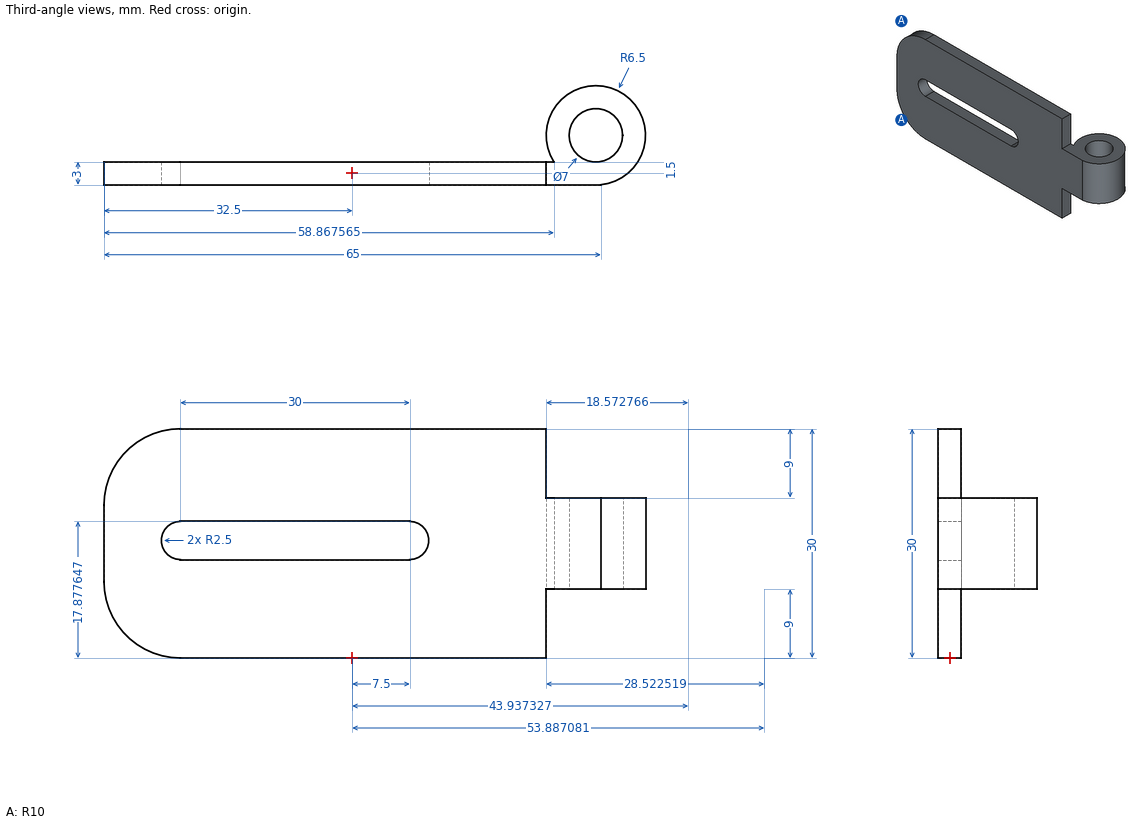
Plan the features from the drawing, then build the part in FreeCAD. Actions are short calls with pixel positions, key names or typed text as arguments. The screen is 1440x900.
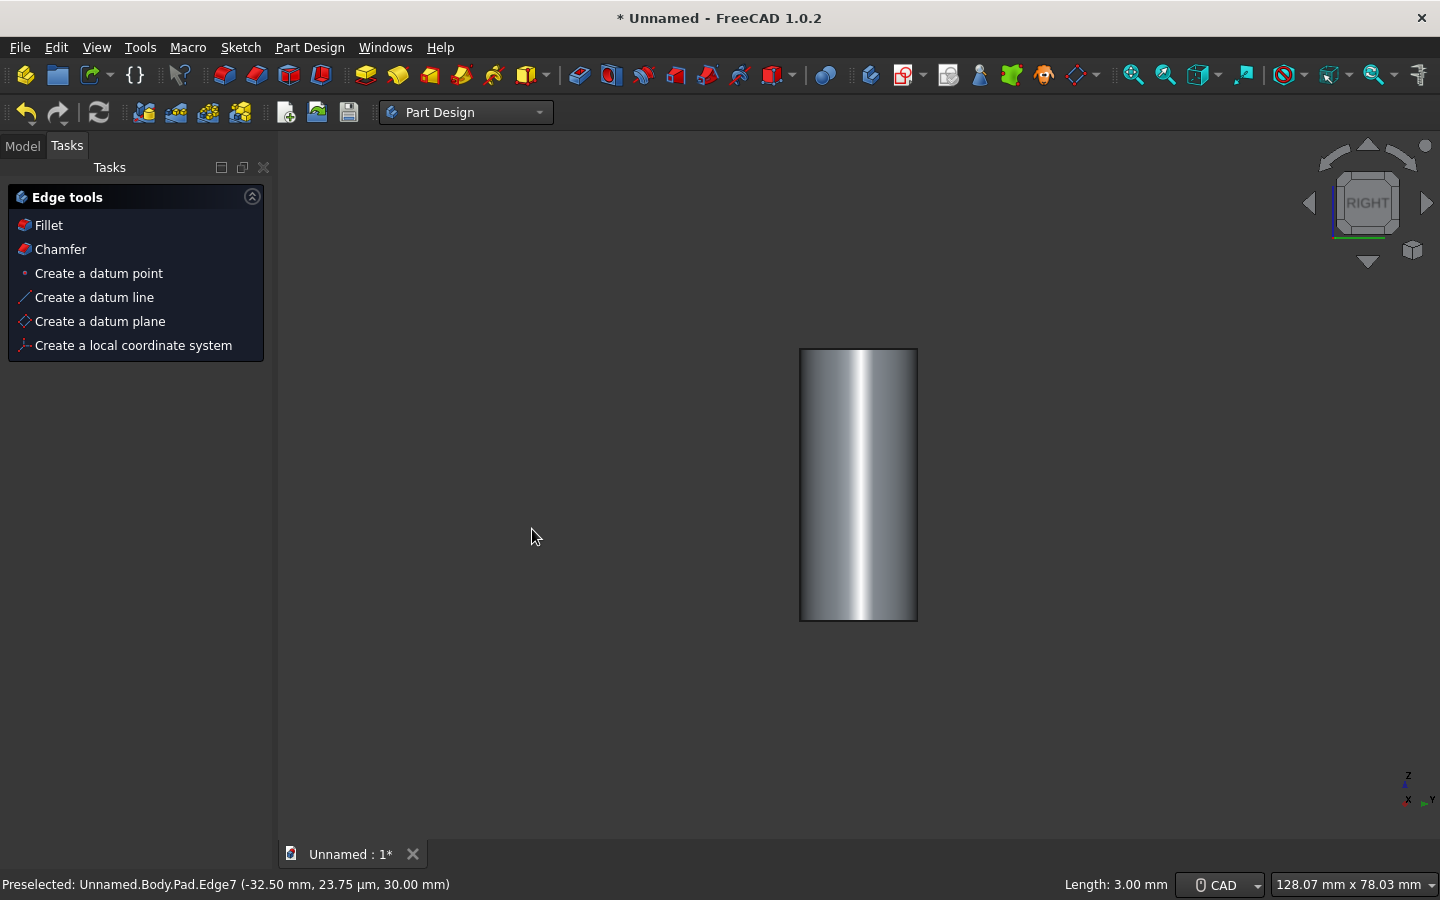
click(1134, 76)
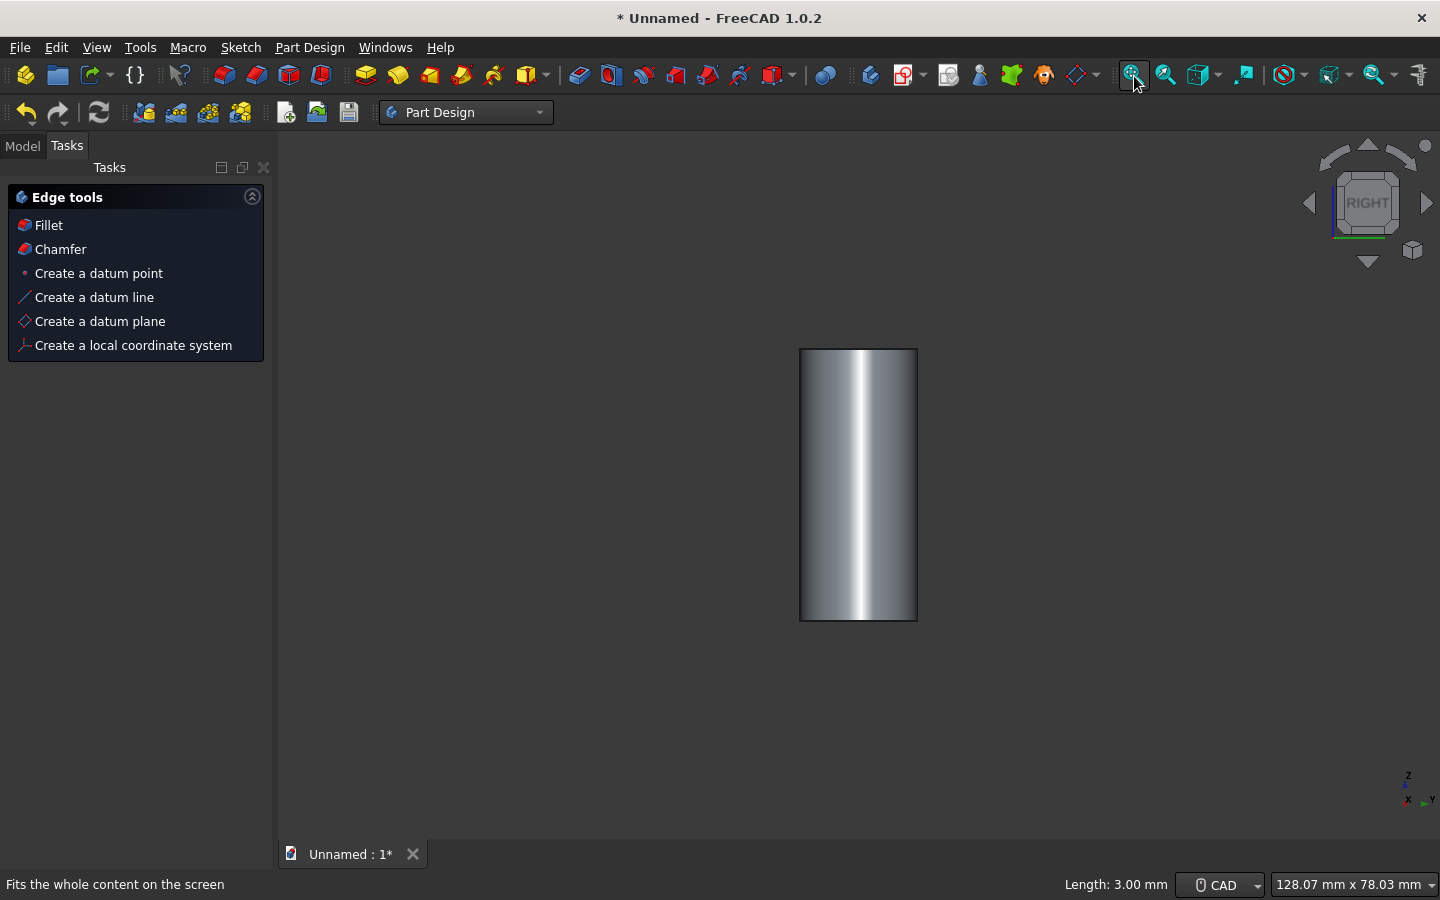
key(5)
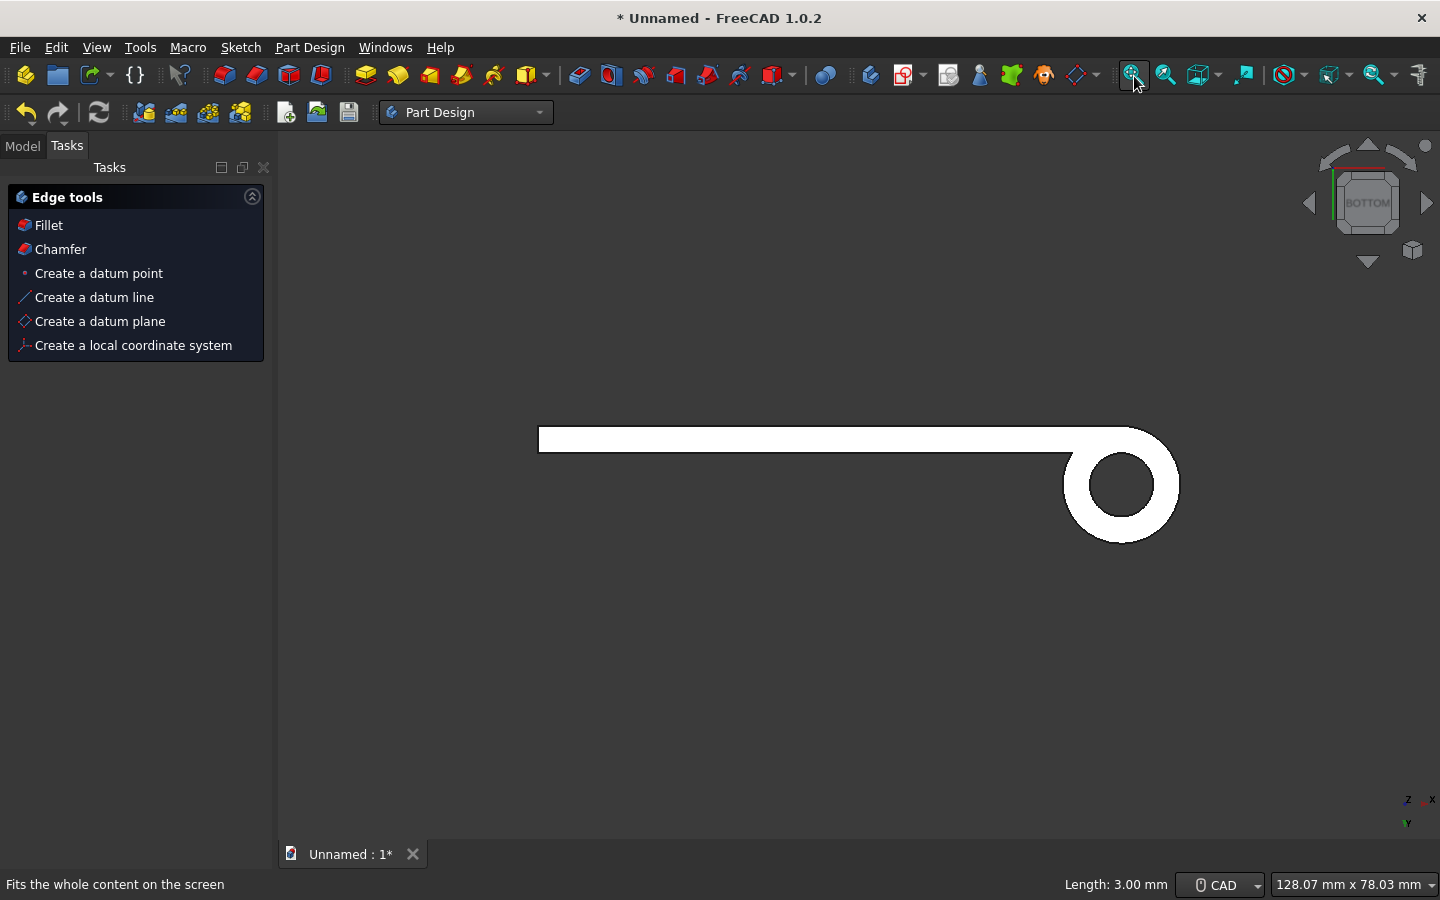
click(538, 439, ctrl)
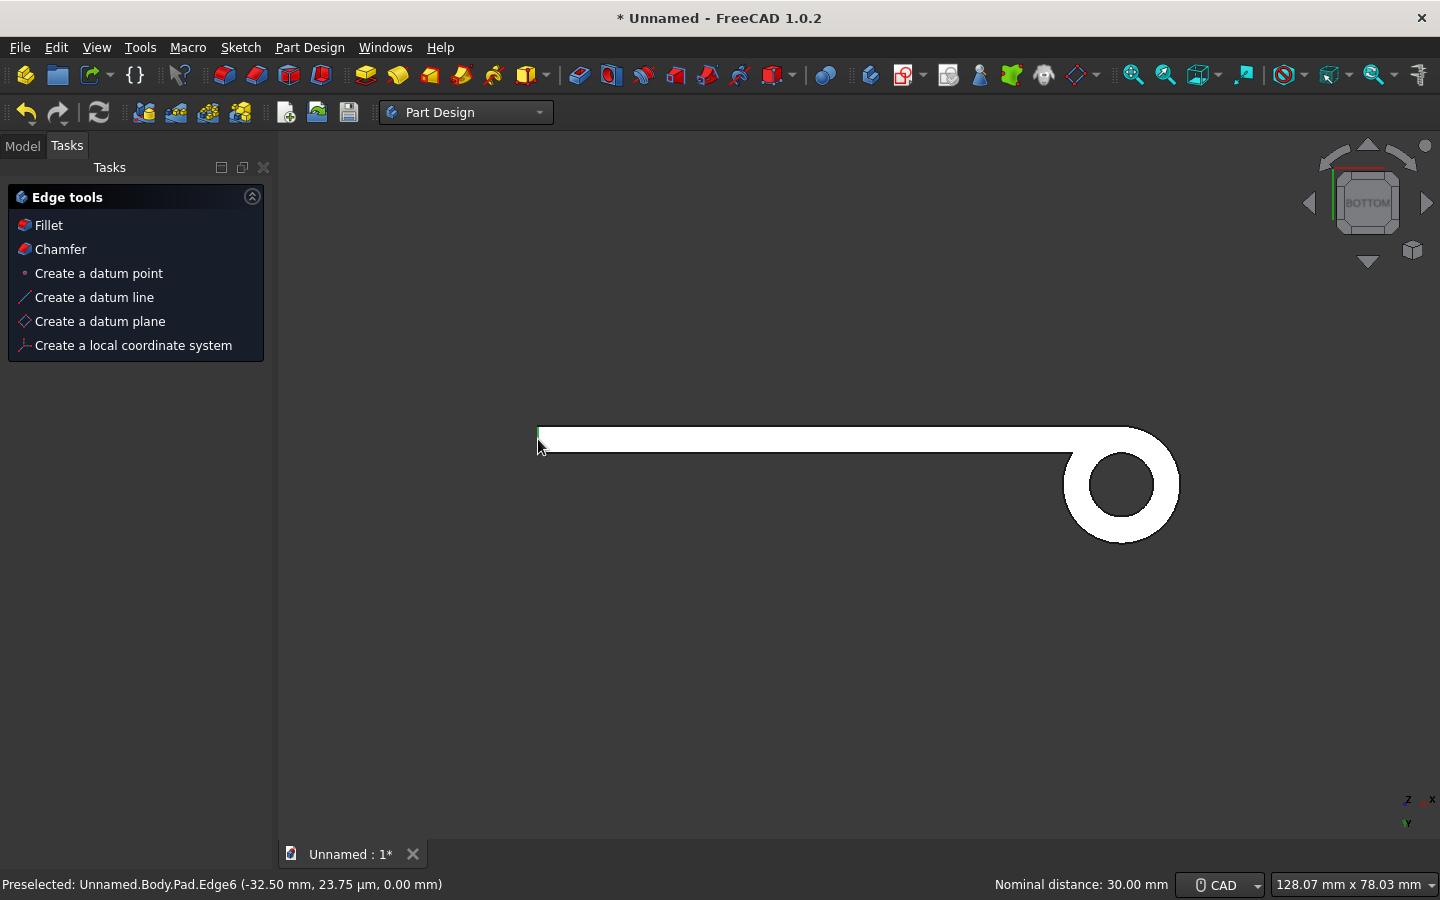
click(226, 76)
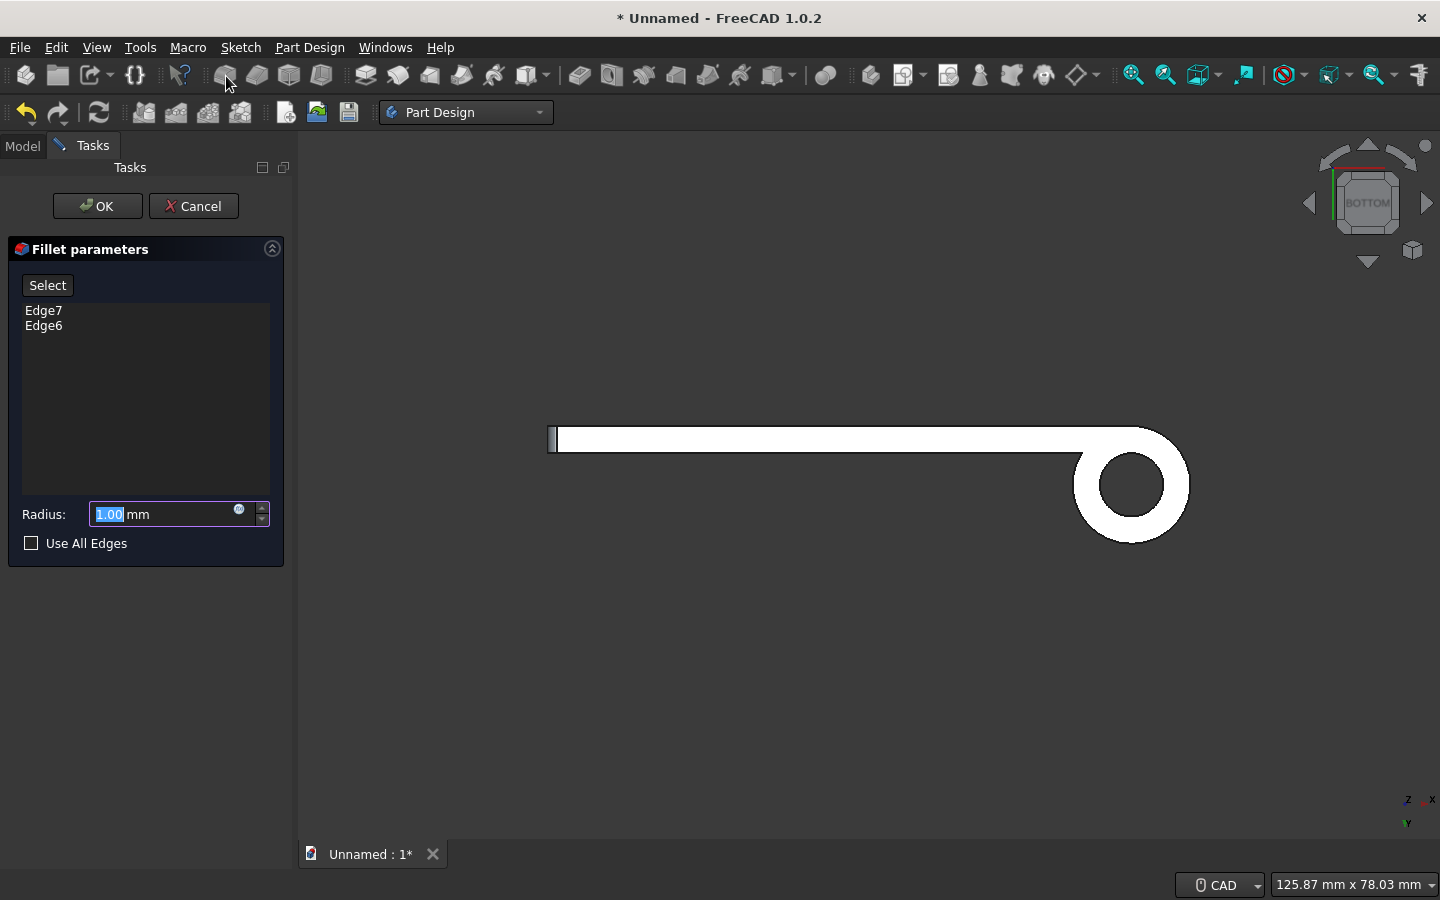
text(10)
key(Tab)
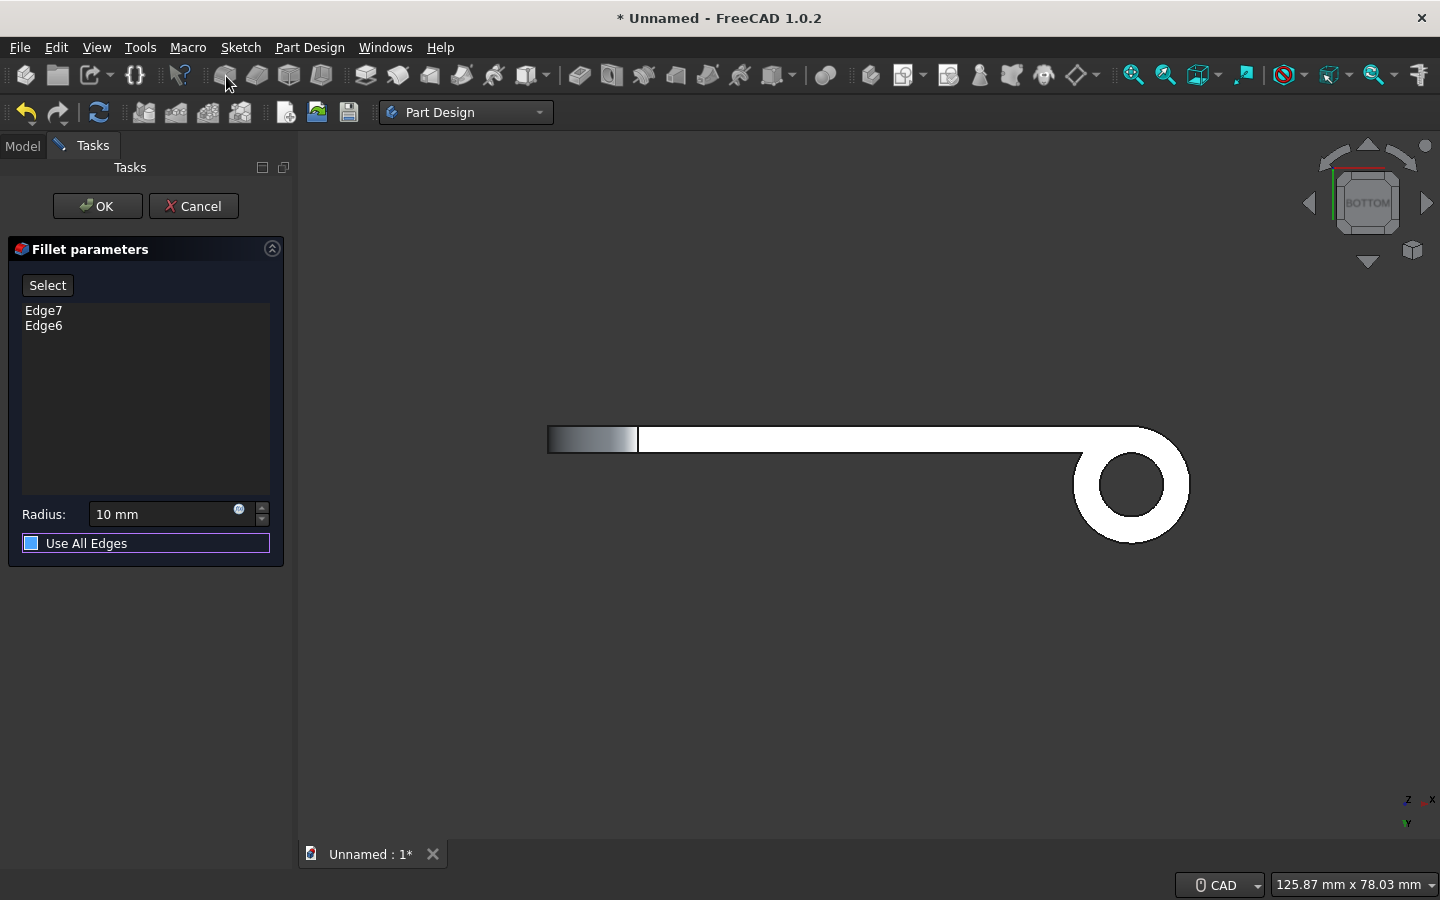
click(98, 206)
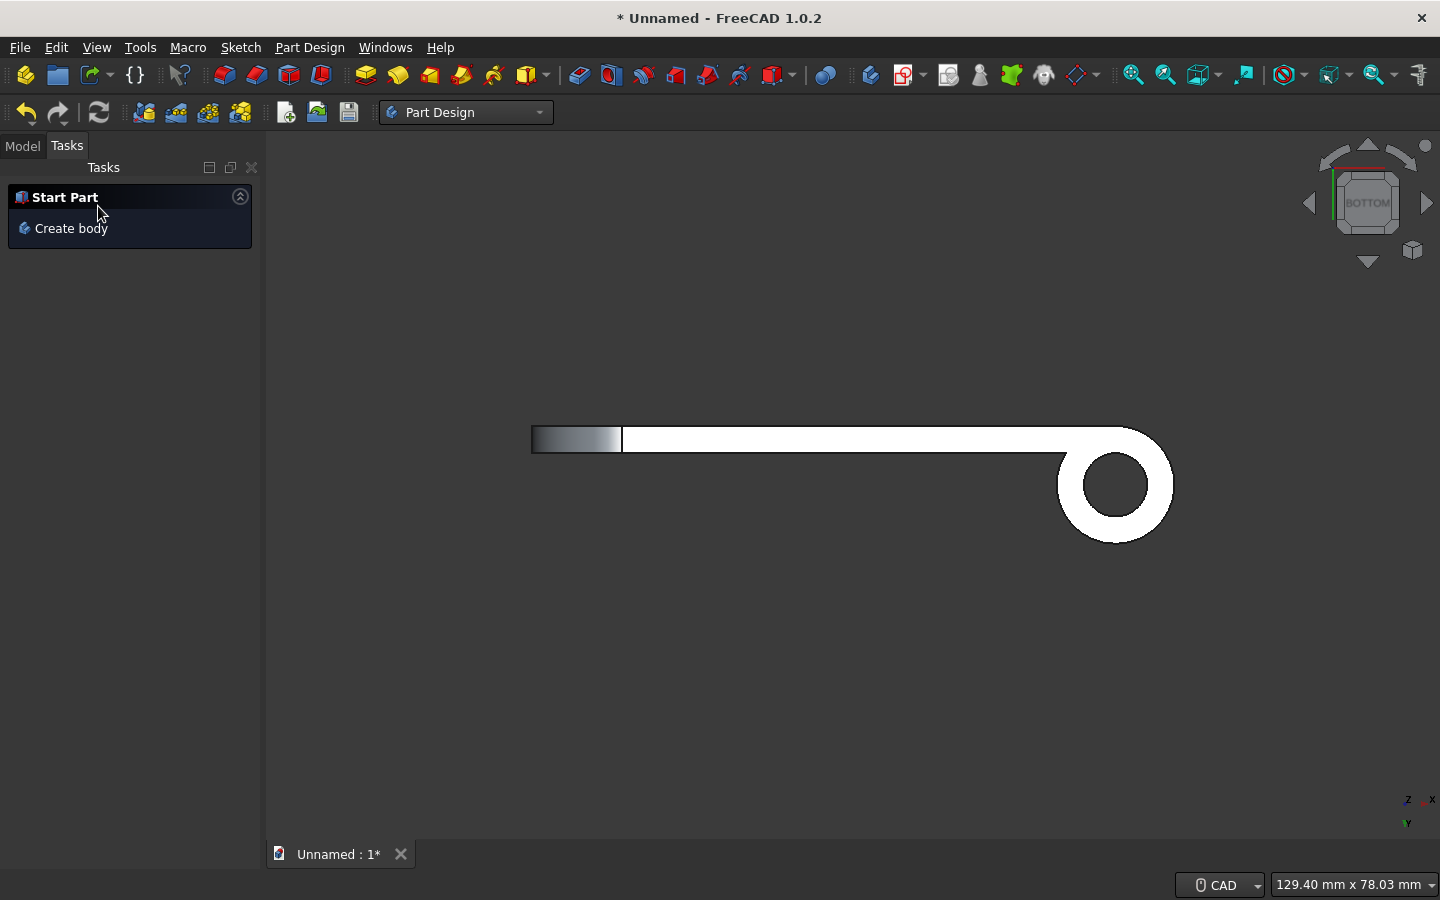
key(4)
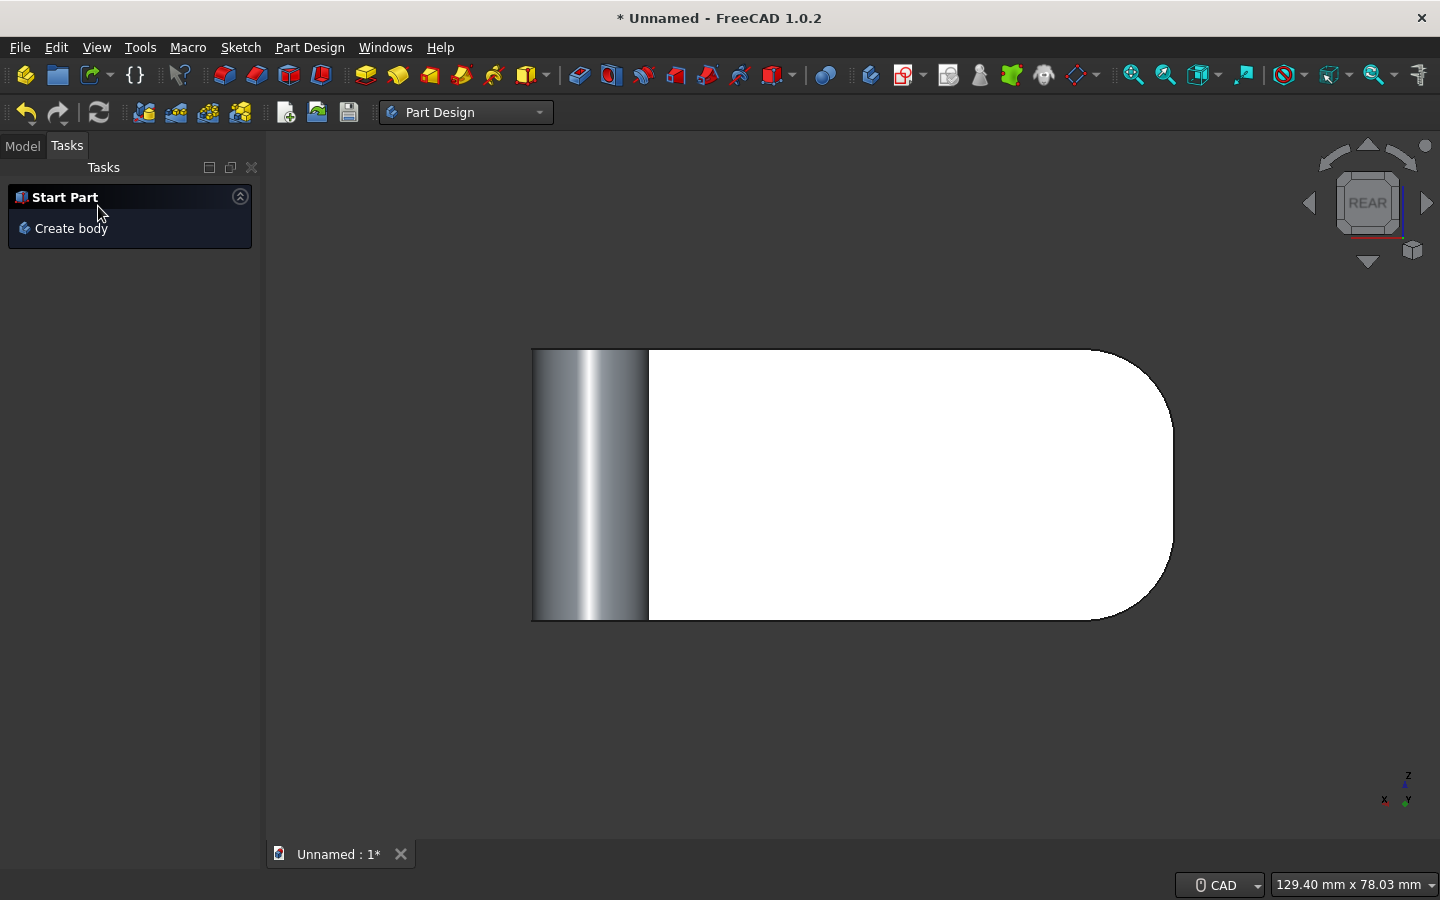
click(831, 484)